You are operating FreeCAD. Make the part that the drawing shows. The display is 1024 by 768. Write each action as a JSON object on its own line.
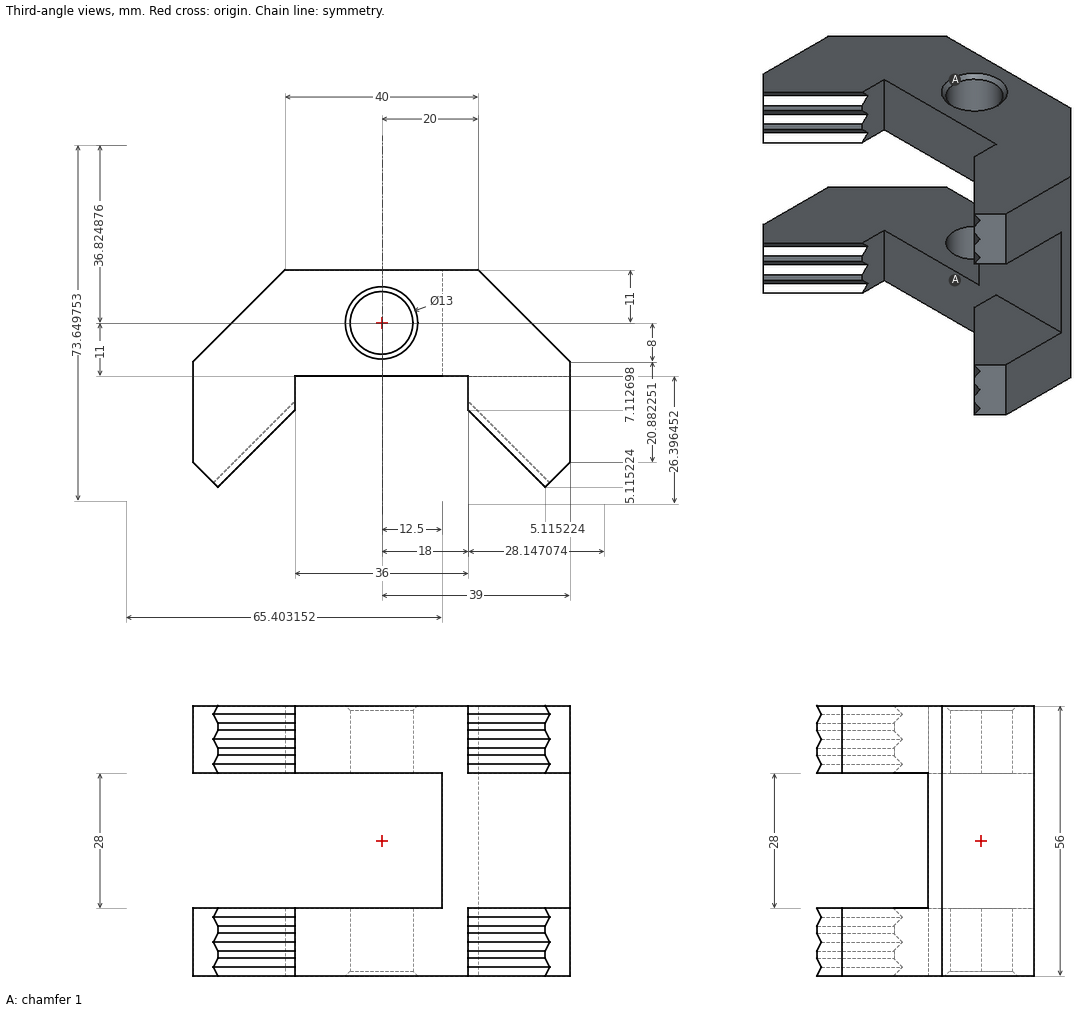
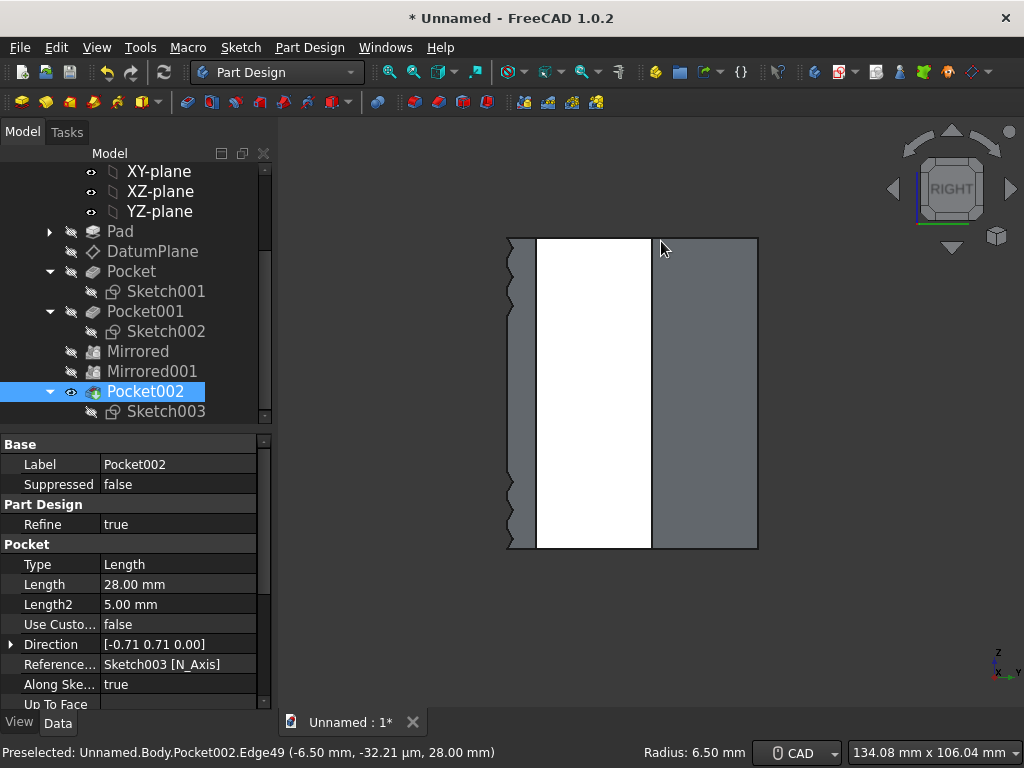
{"action": "key", "text": "5"}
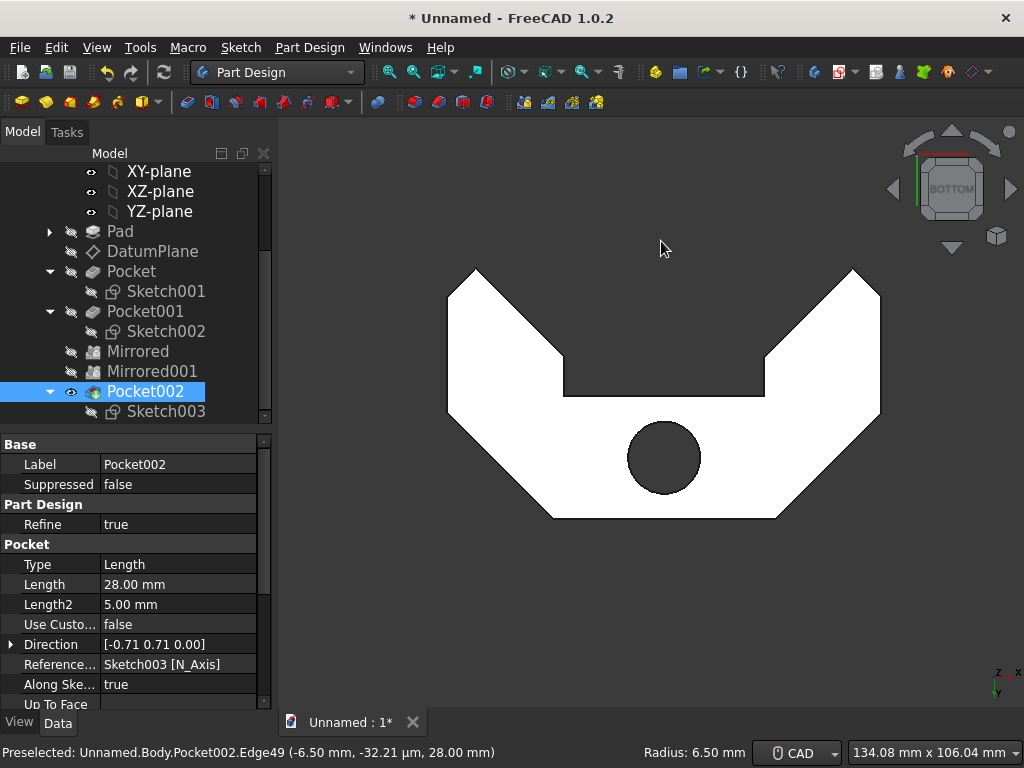
{"action": "left_click", "coordinate": [628, 457], "text": "ctrl"}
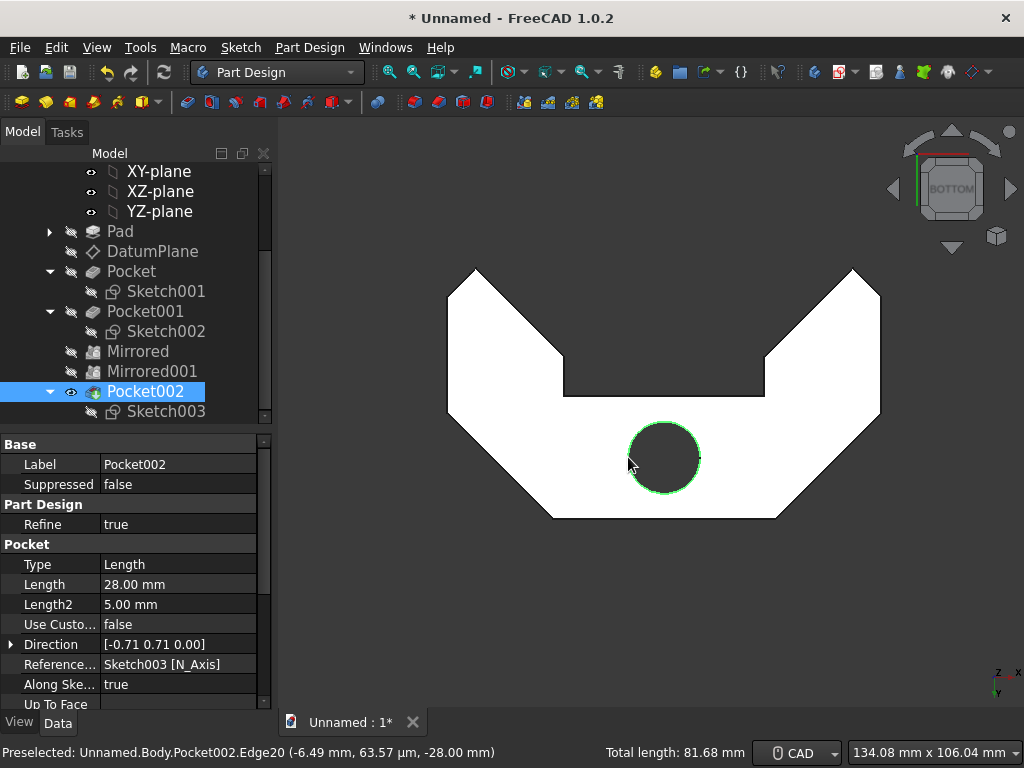
{"action": "left_click", "coordinate": [440, 102]}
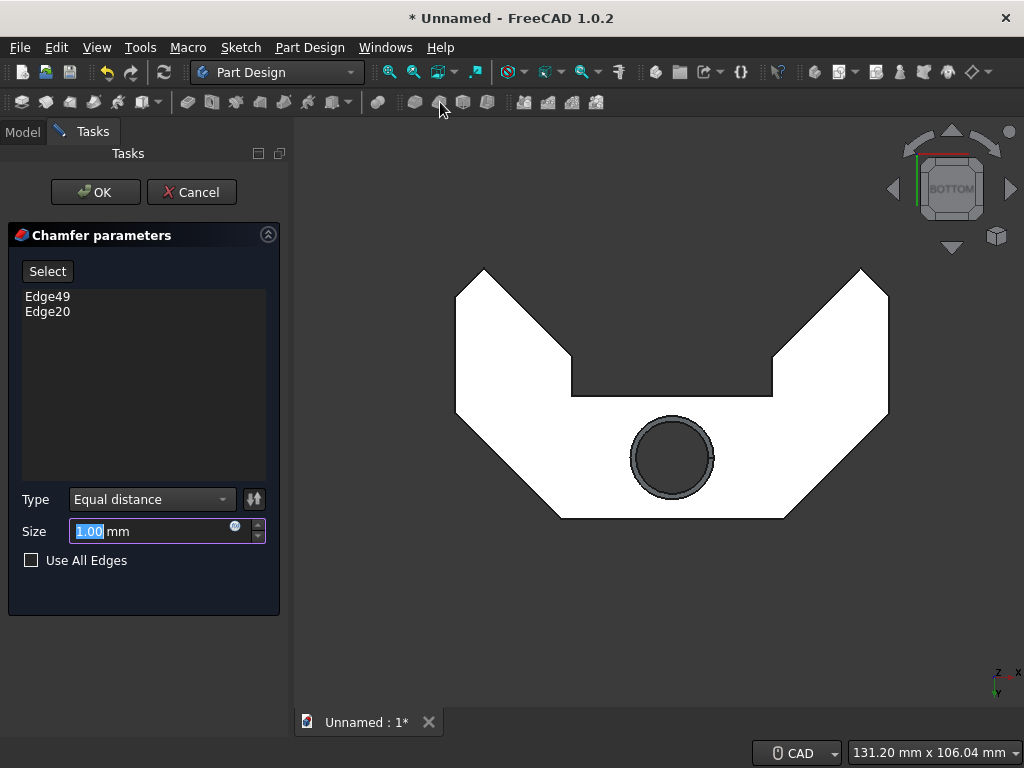
{"action": "type", "text": "1"}
{"action": "key", "text": "Tab"}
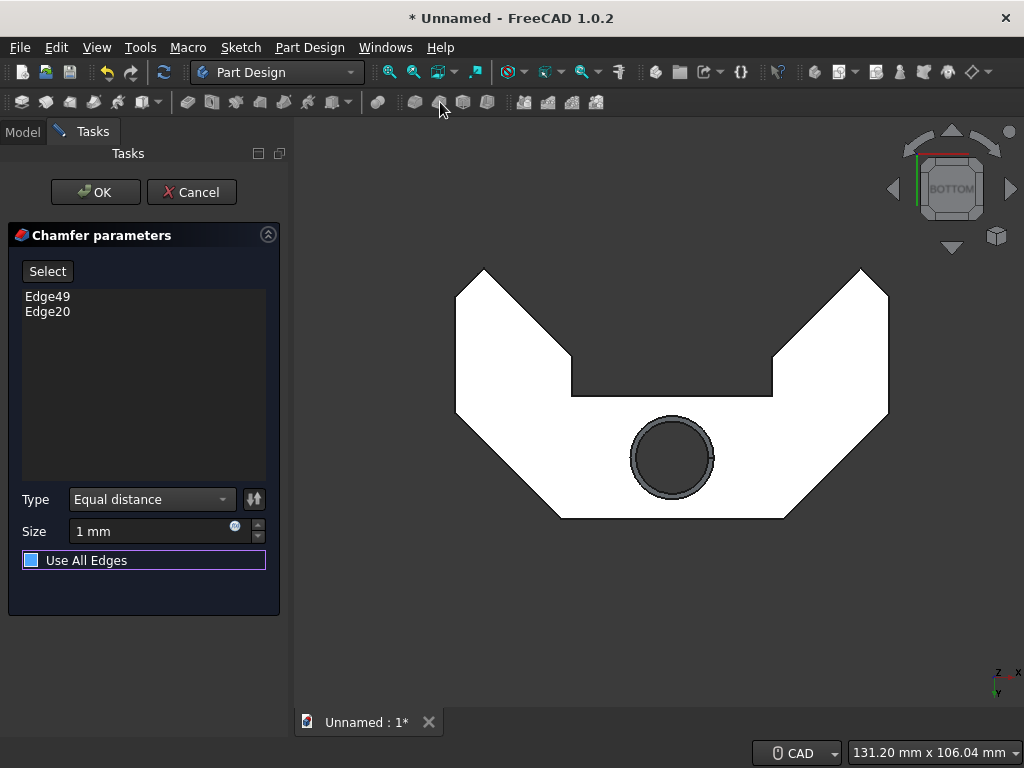
{"action": "left_click", "coordinate": [96, 192]}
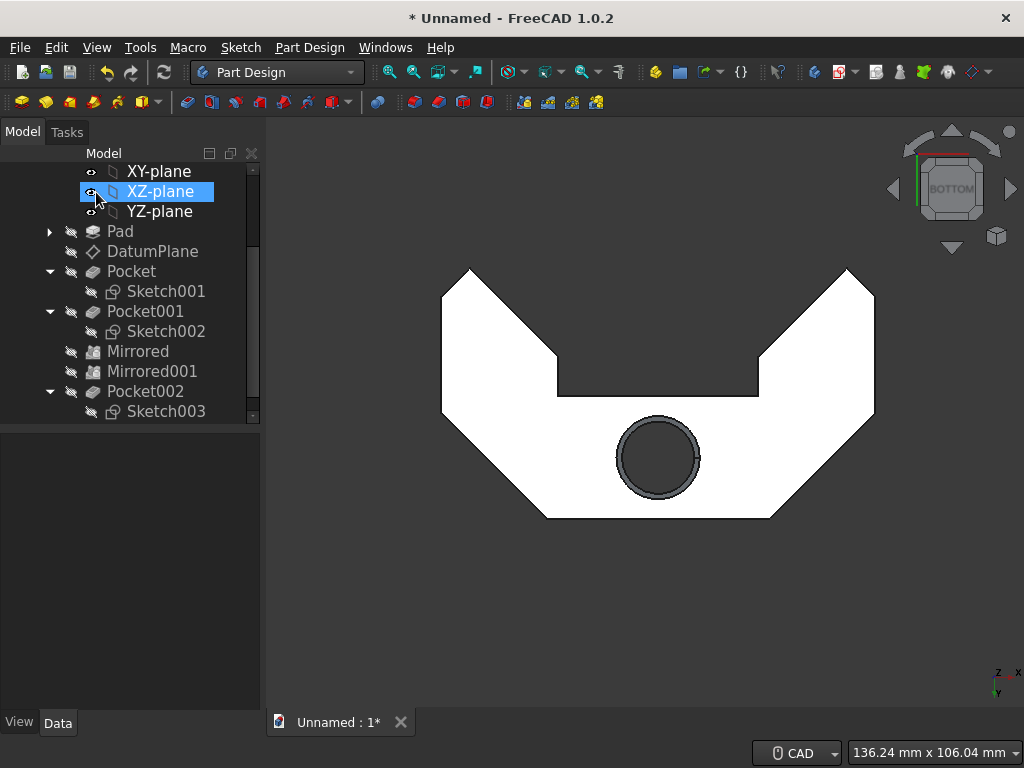
{"action": "scroll", "coordinate": [160, 287], "scroll_direction": "down", "scroll_amount": 3}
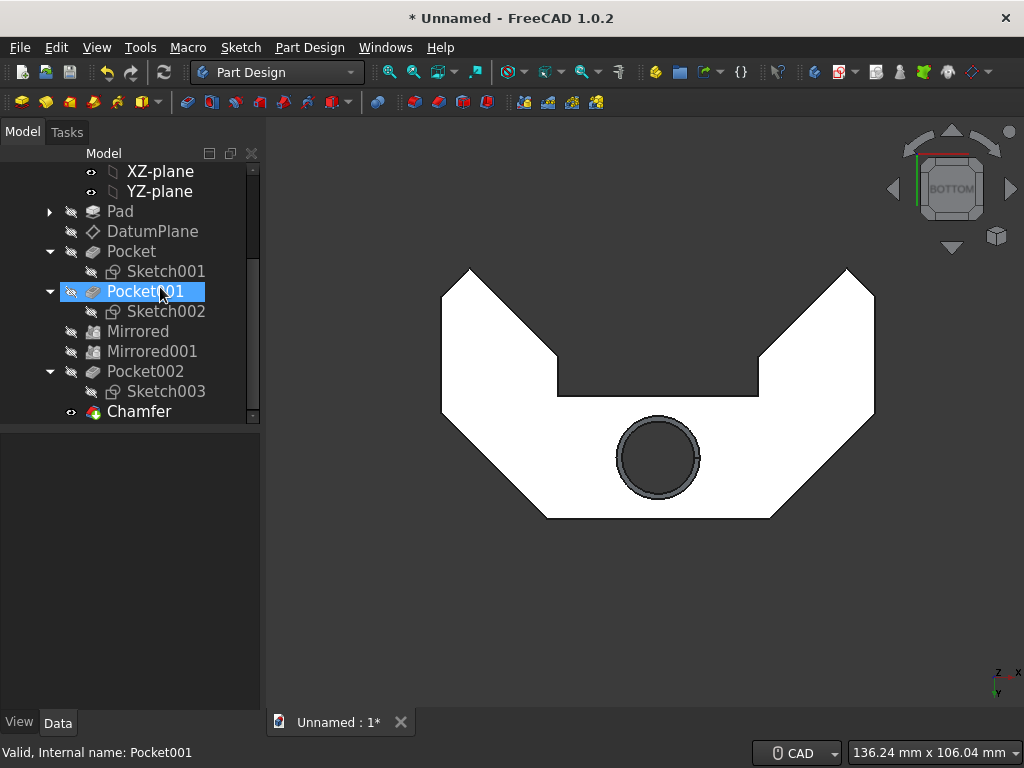
{"action": "scroll", "coordinate": [160, 287], "scroll_direction": "up", "scroll_amount": 15}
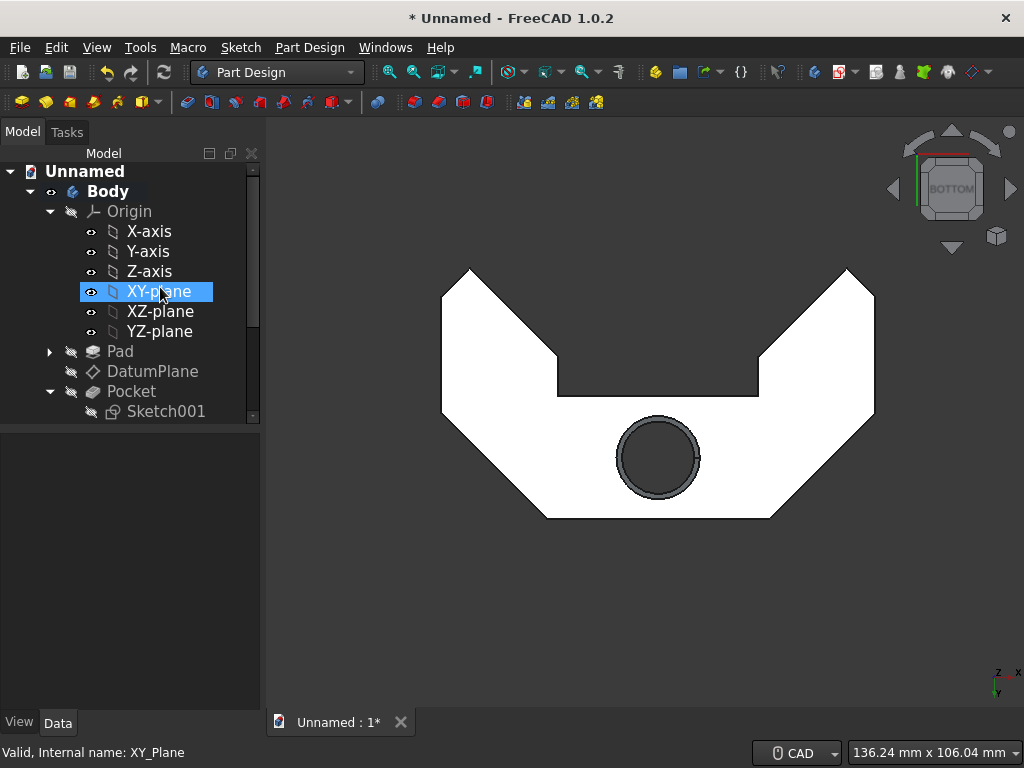
{"action": "left_click", "coordinate": [136, 292]}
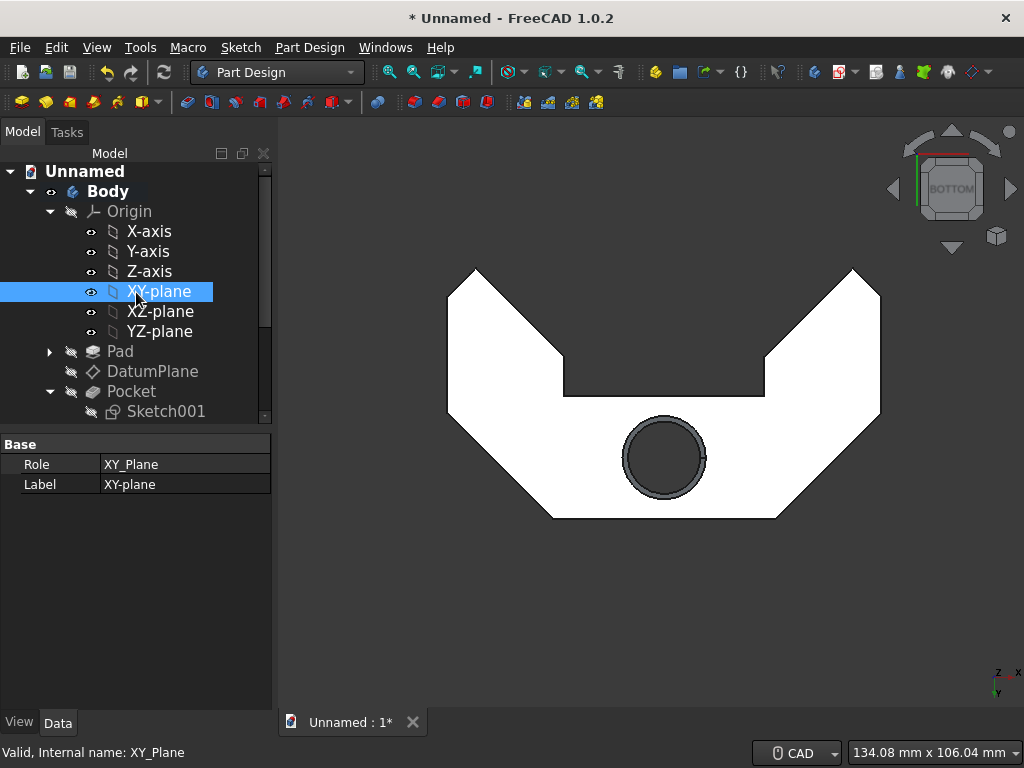
{"action": "left_click", "coordinate": [972, 72]}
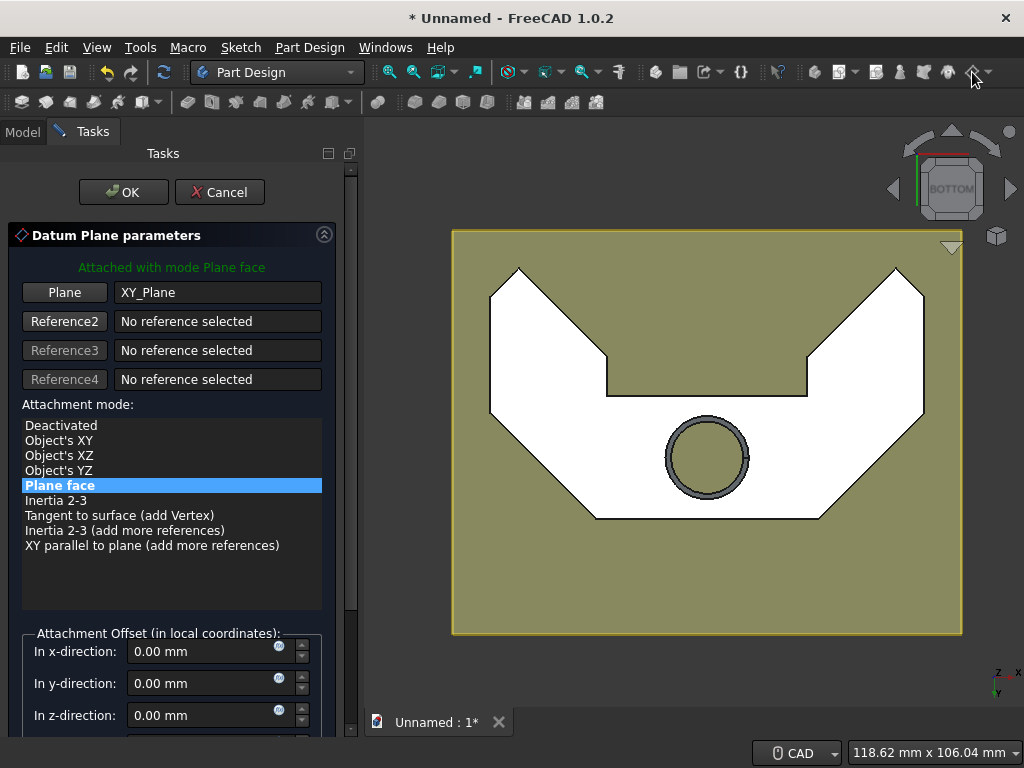
{"action": "triple_click", "coordinate": [210, 715]}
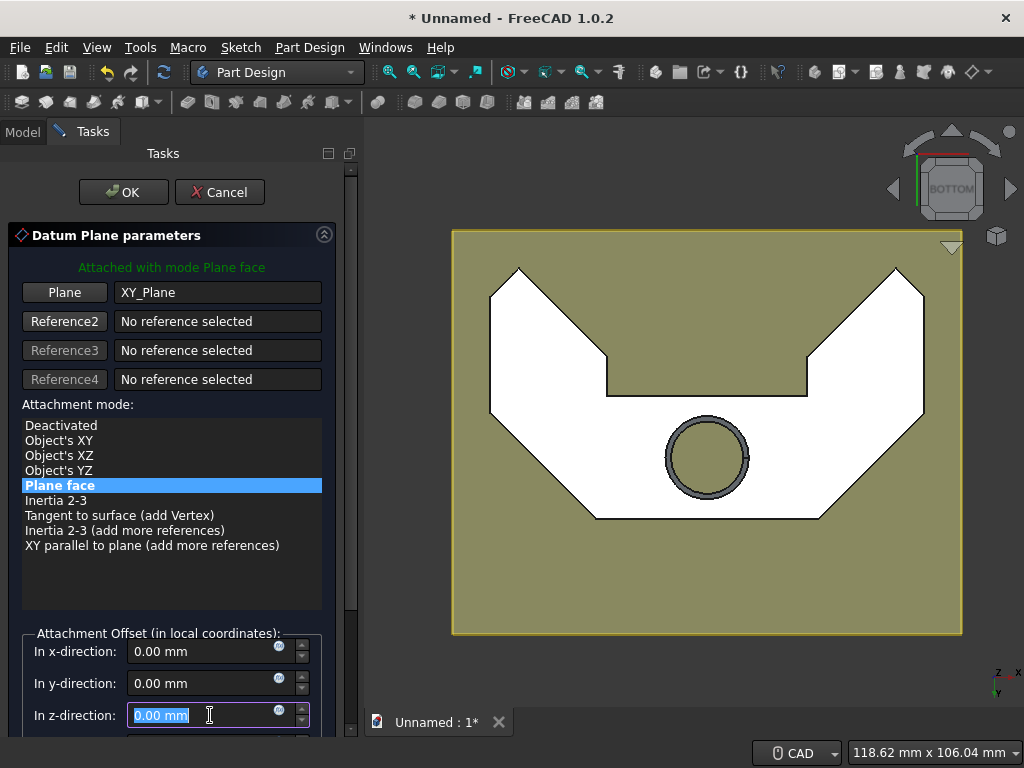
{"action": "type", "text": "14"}
{"action": "key", "text": "Tab"}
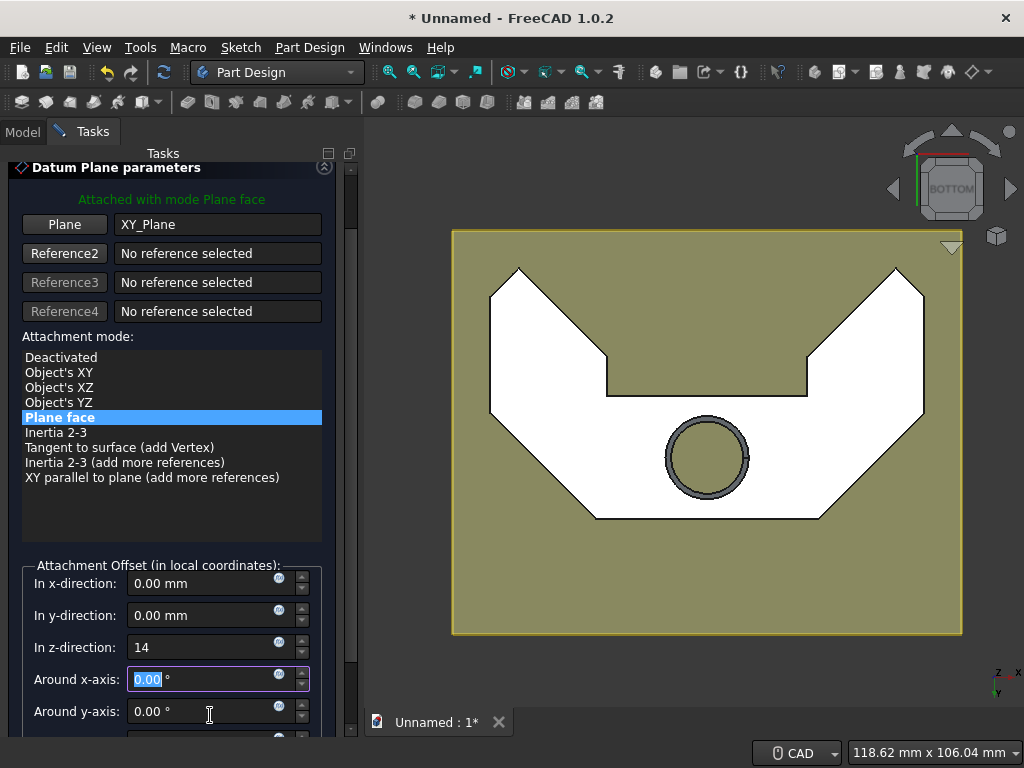
{"action": "scroll", "coordinate": [351, 450], "scroll_direction": "up", "scroll_amount": 2}